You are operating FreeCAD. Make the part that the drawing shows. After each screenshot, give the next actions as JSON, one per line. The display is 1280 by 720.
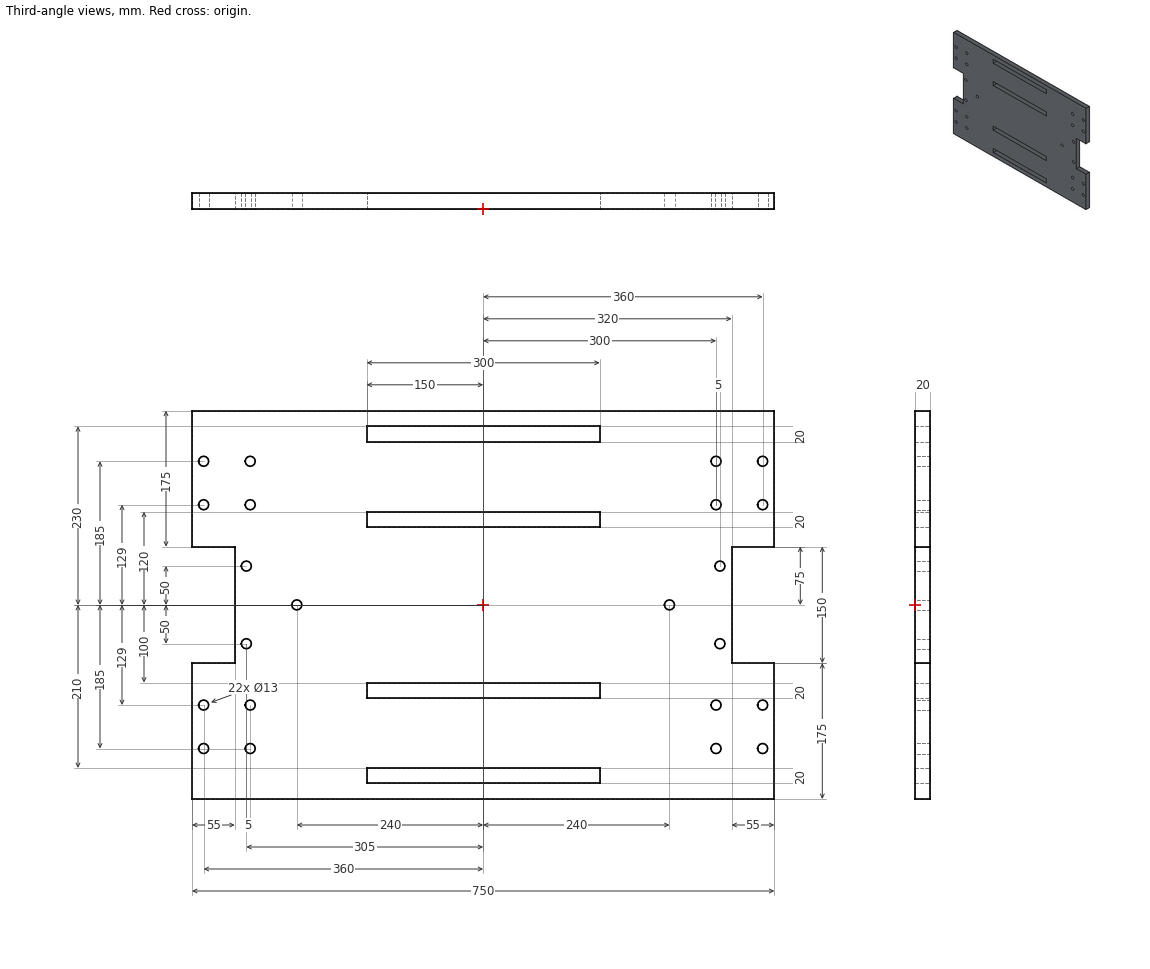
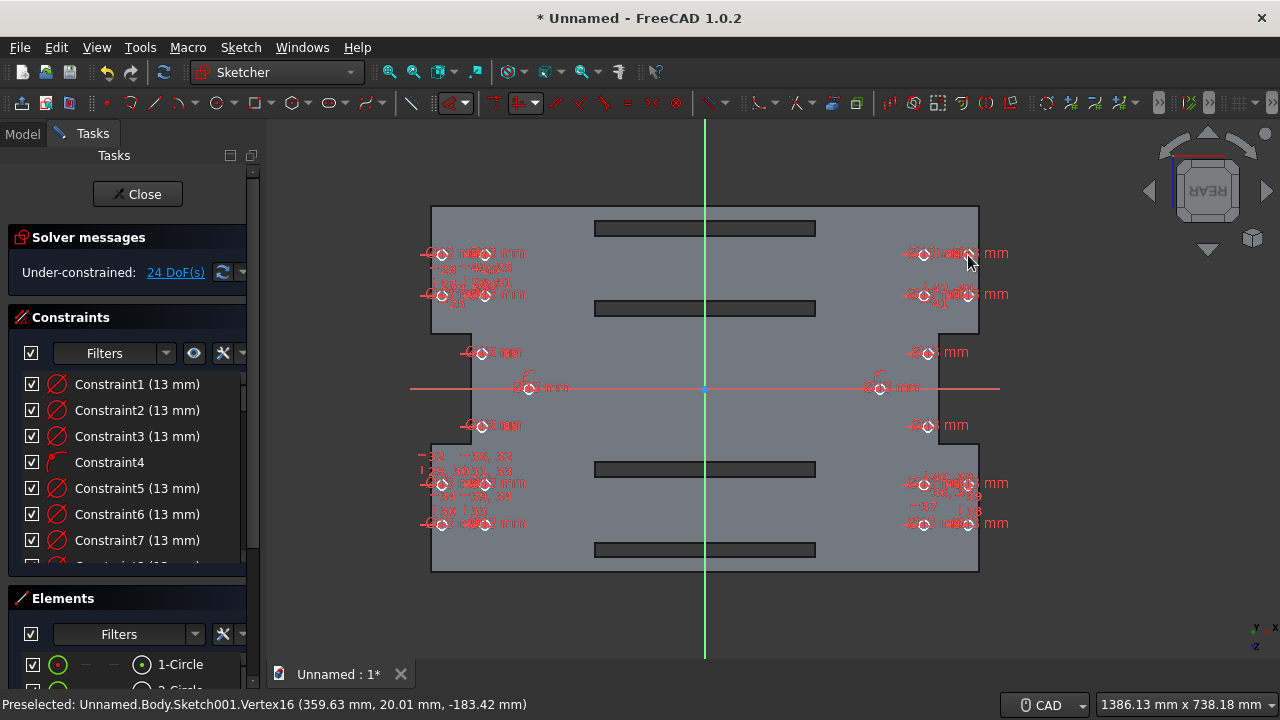
{"action": "key", "text": "h"}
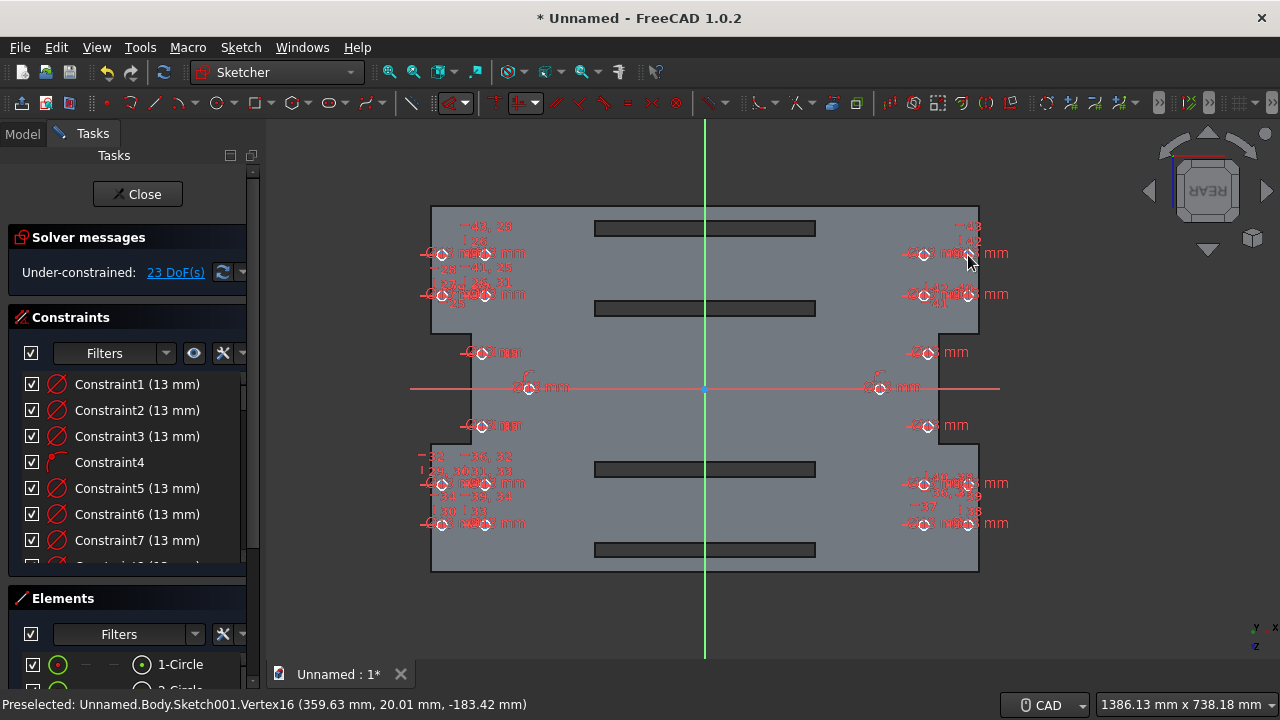
{"action": "left_click", "coordinate": [924, 485]}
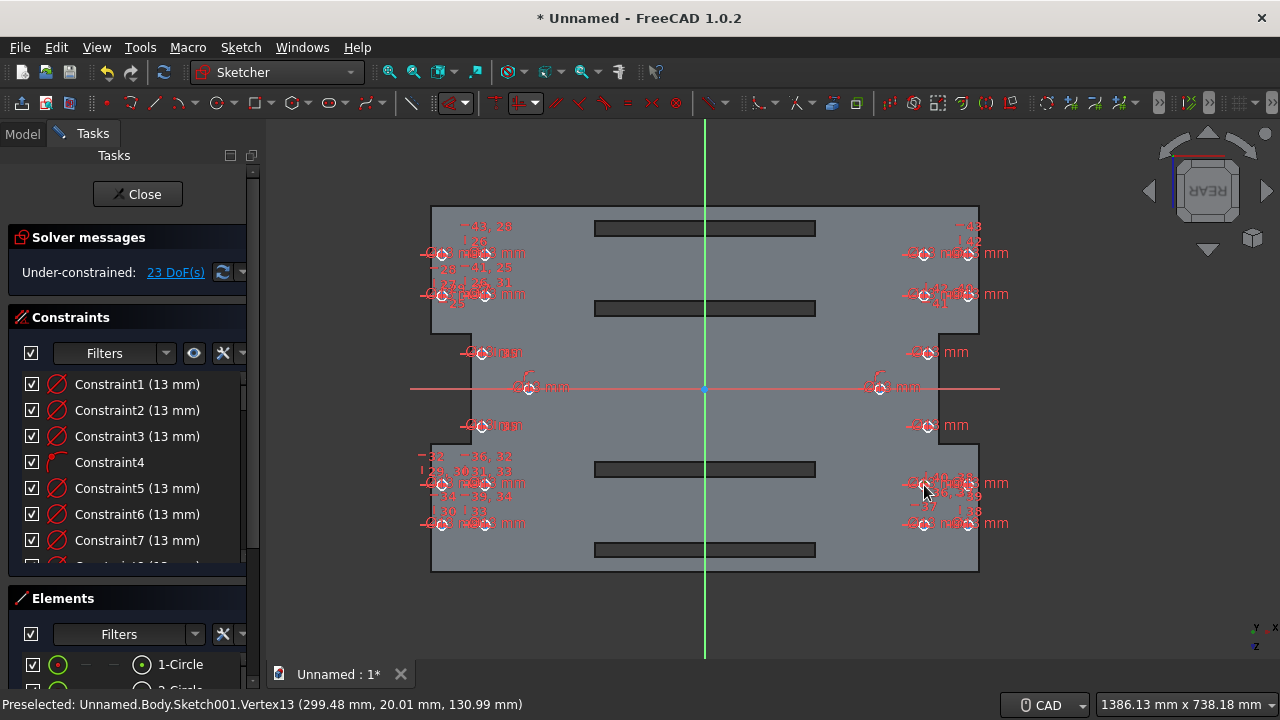
{"action": "left_click", "coordinate": [924, 296]}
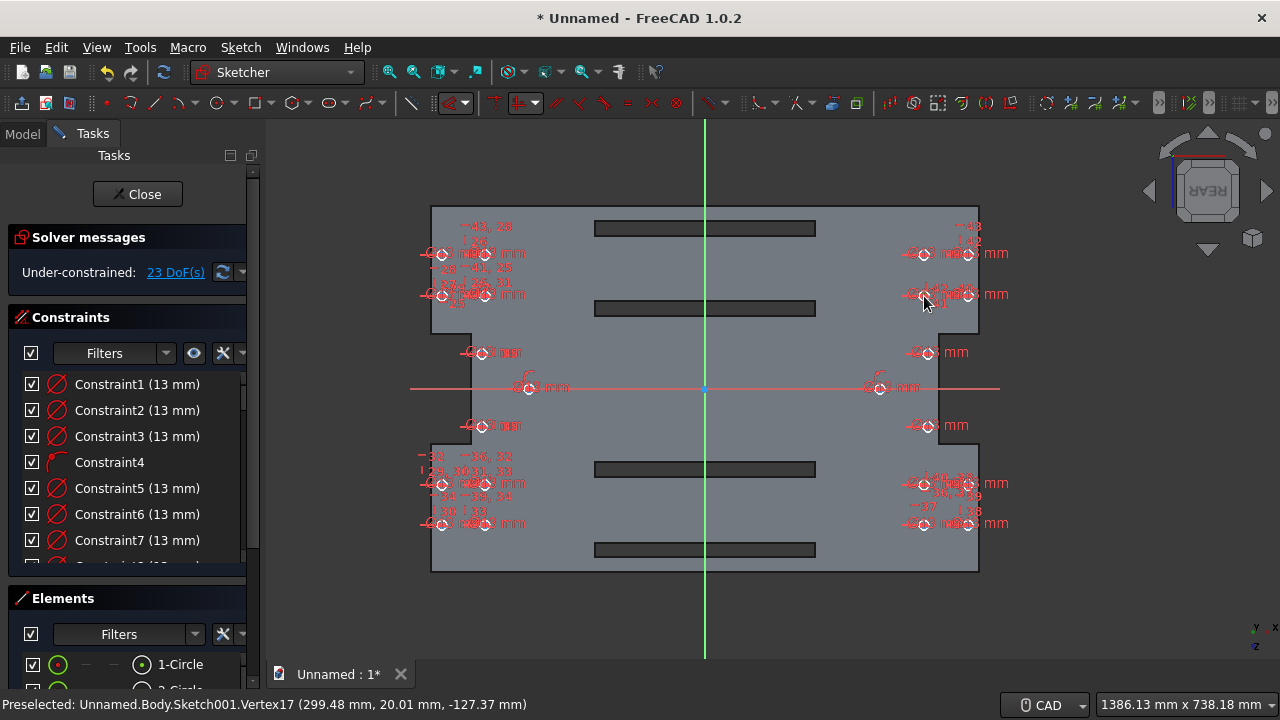
{"action": "key", "text": "v"}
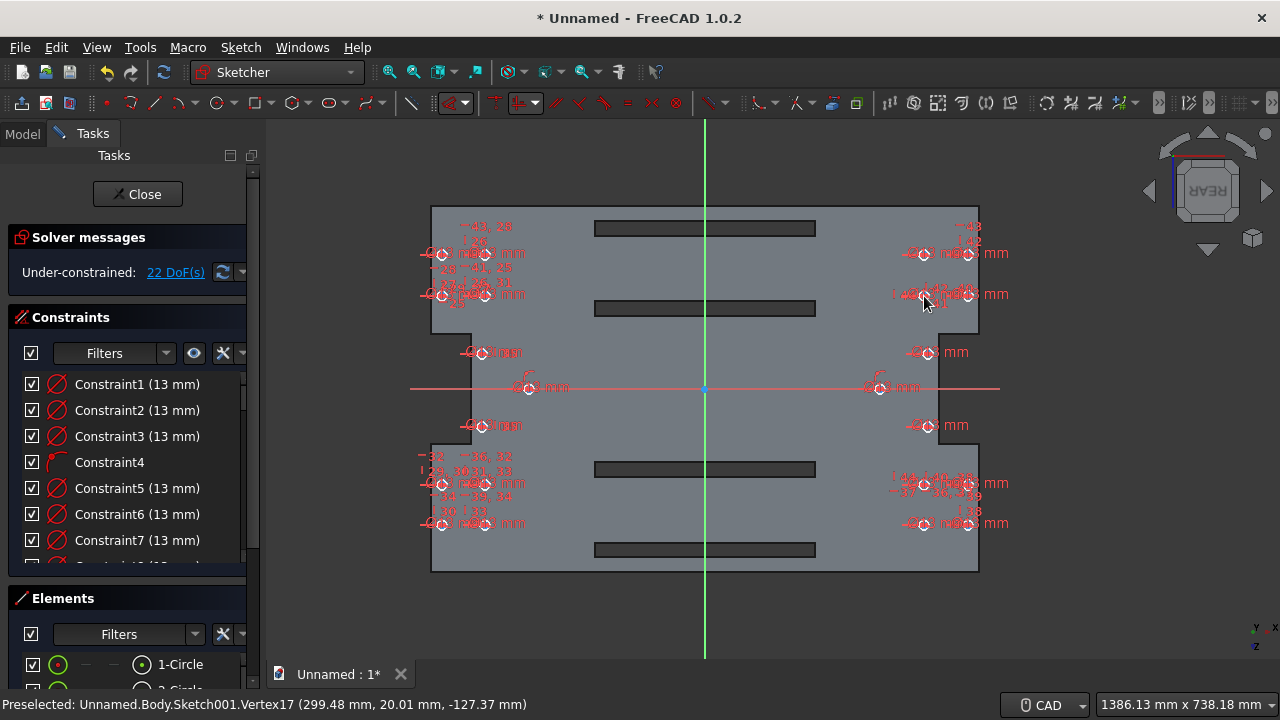
{"action": "left_click", "coordinate": [968, 296]}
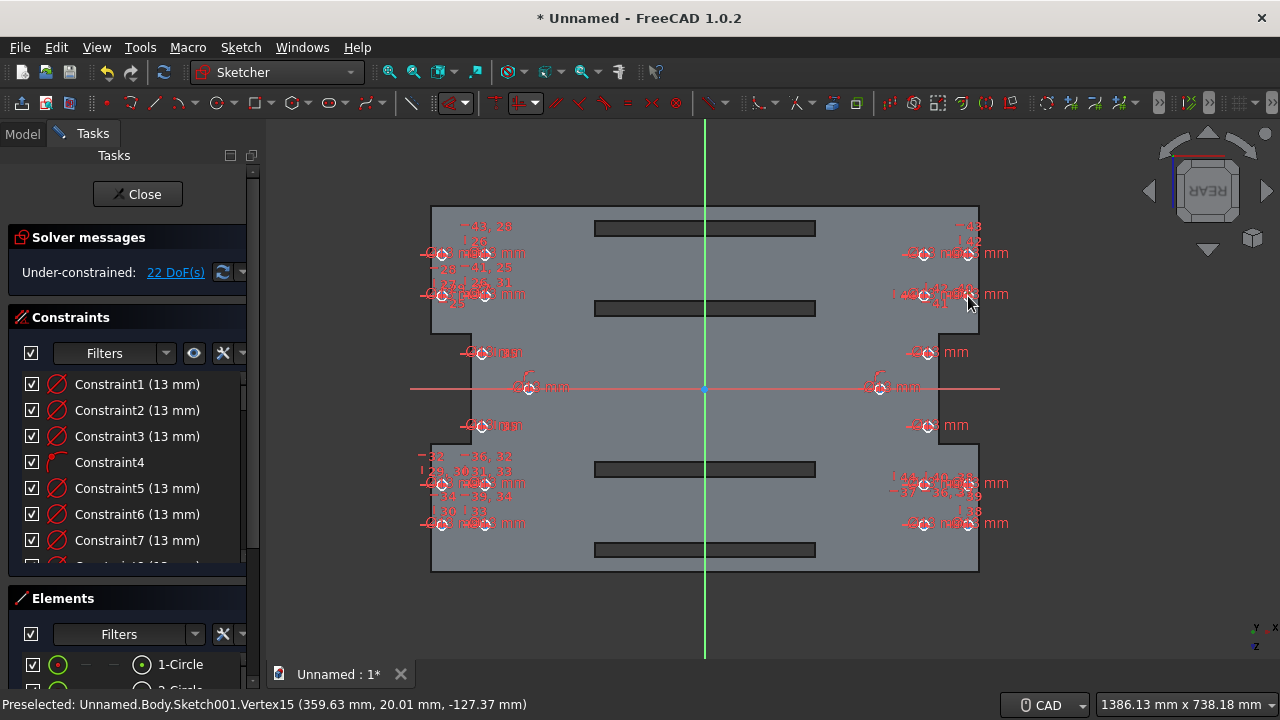
{"action": "left_click", "coordinate": [924, 296]}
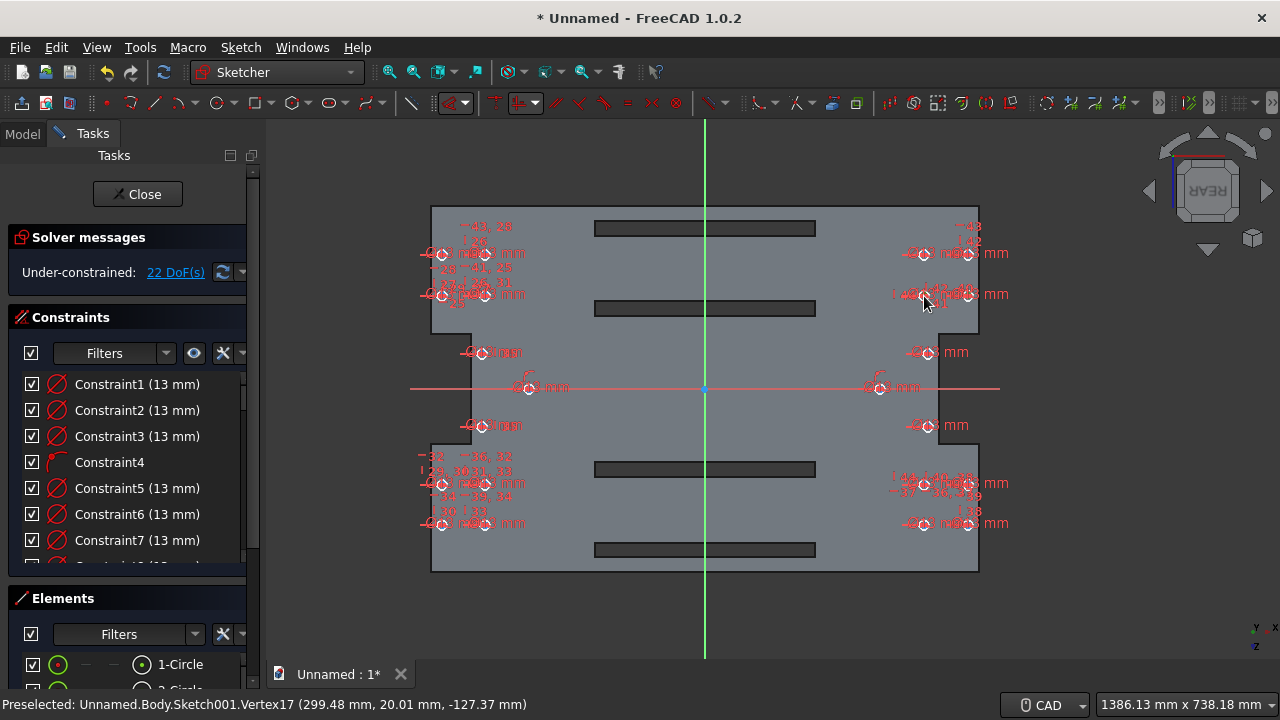
{"action": "key", "text": "h"}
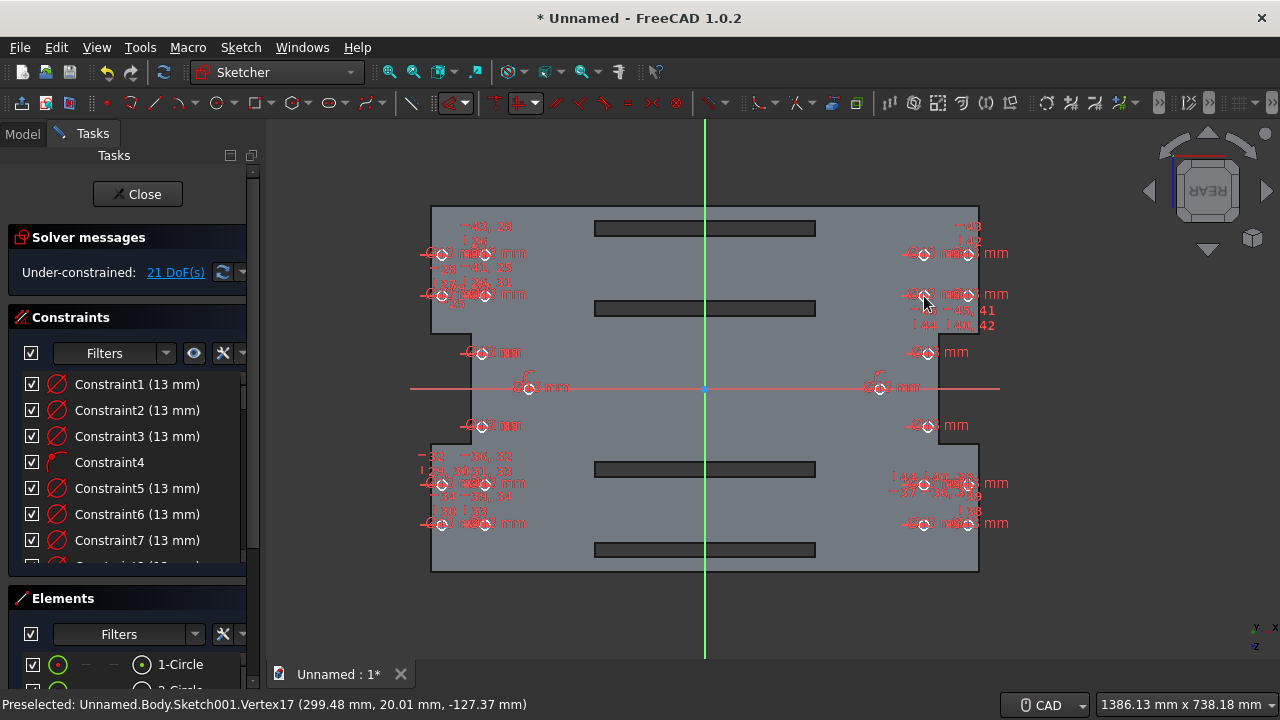
{"action": "left_click", "coordinate": [924, 485]}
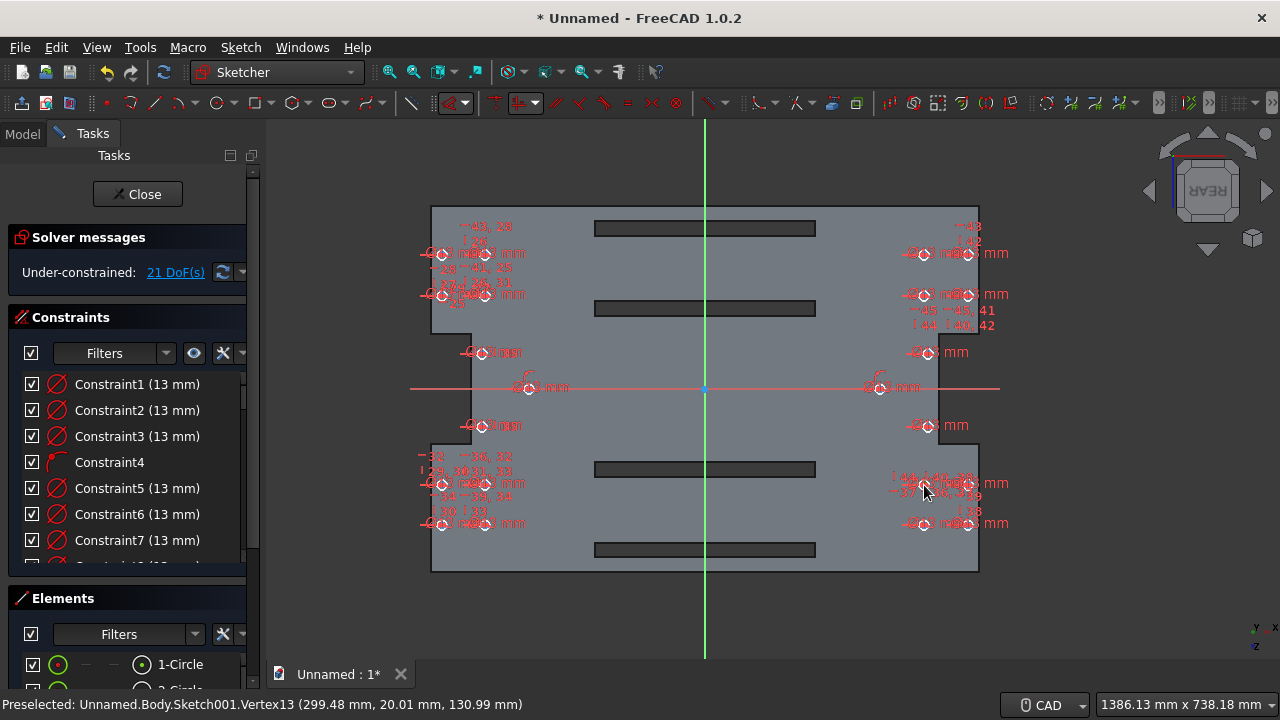
{"action": "left_click", "coordinate": [924, 525]}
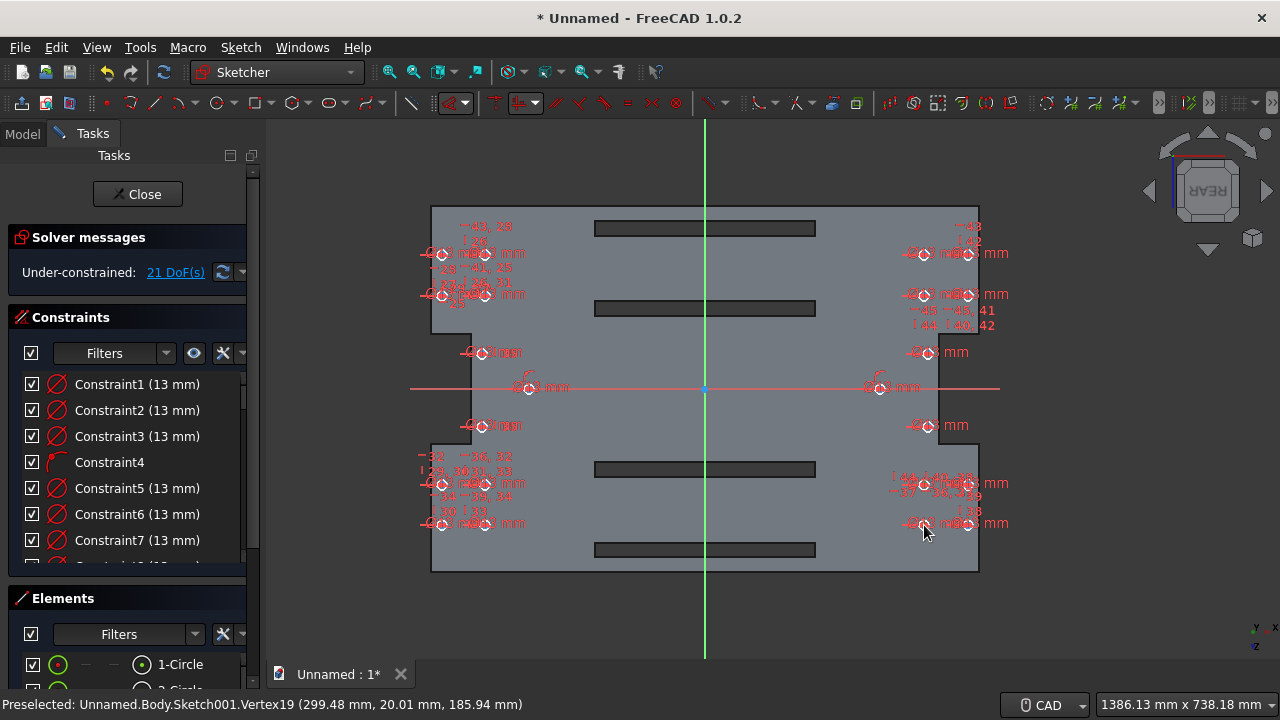
{"action": "key", "text": "v"}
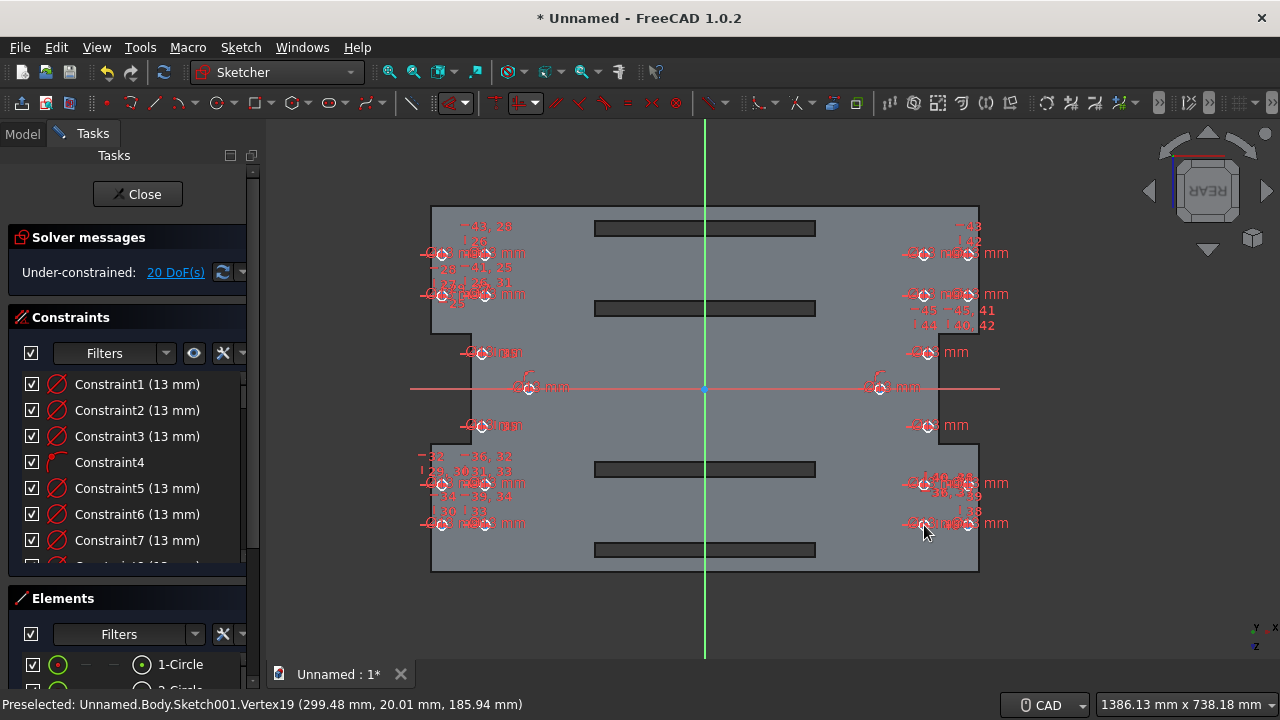
{"action": "left_click", "coordinate": [968, 525]}